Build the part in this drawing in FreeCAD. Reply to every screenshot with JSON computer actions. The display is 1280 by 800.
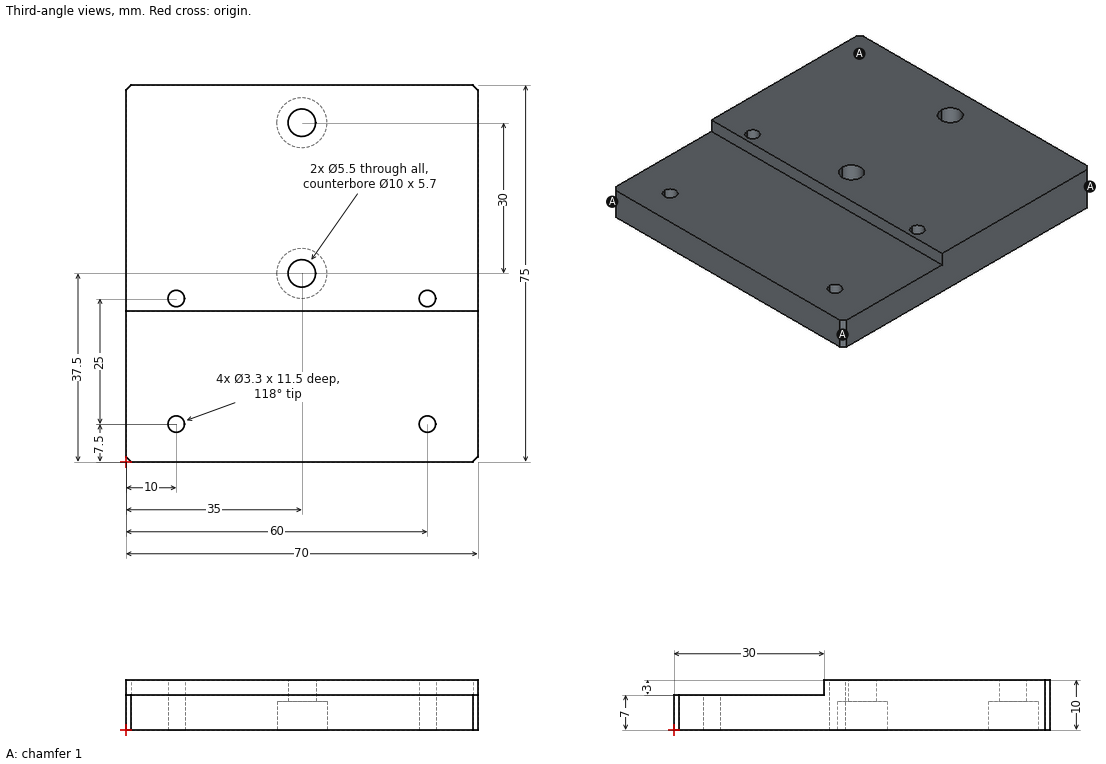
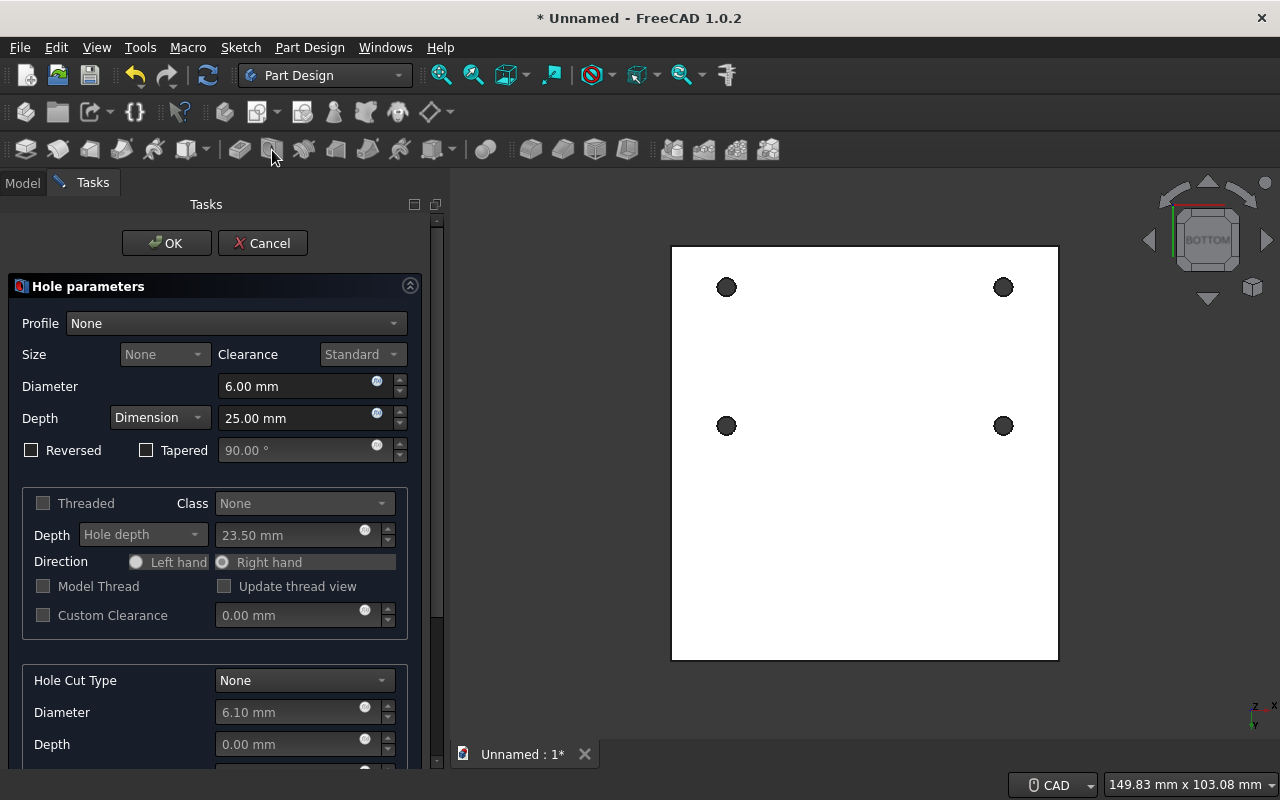
{"action": "triple_click", "coordinate": [305, 386]}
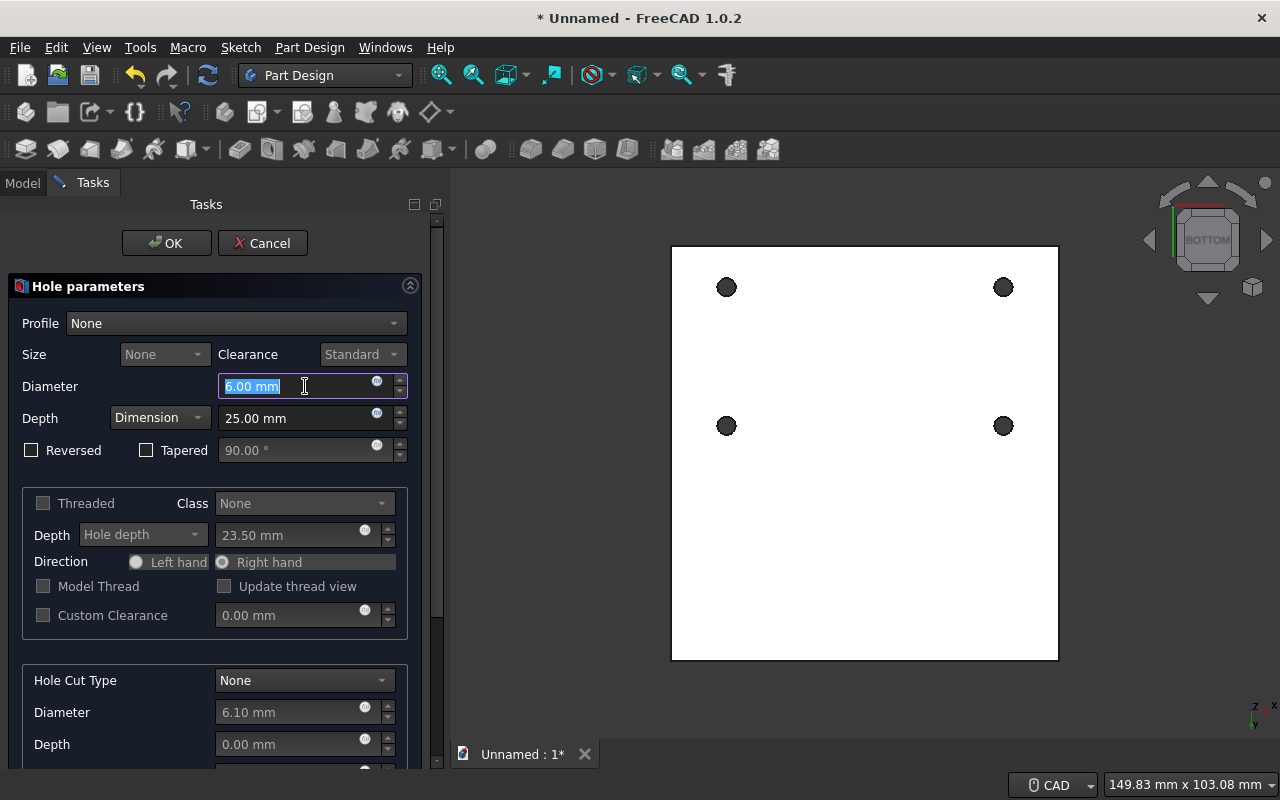
{"action": "type", "text": "5.5"}
{"action": "key", "text": "Tab"}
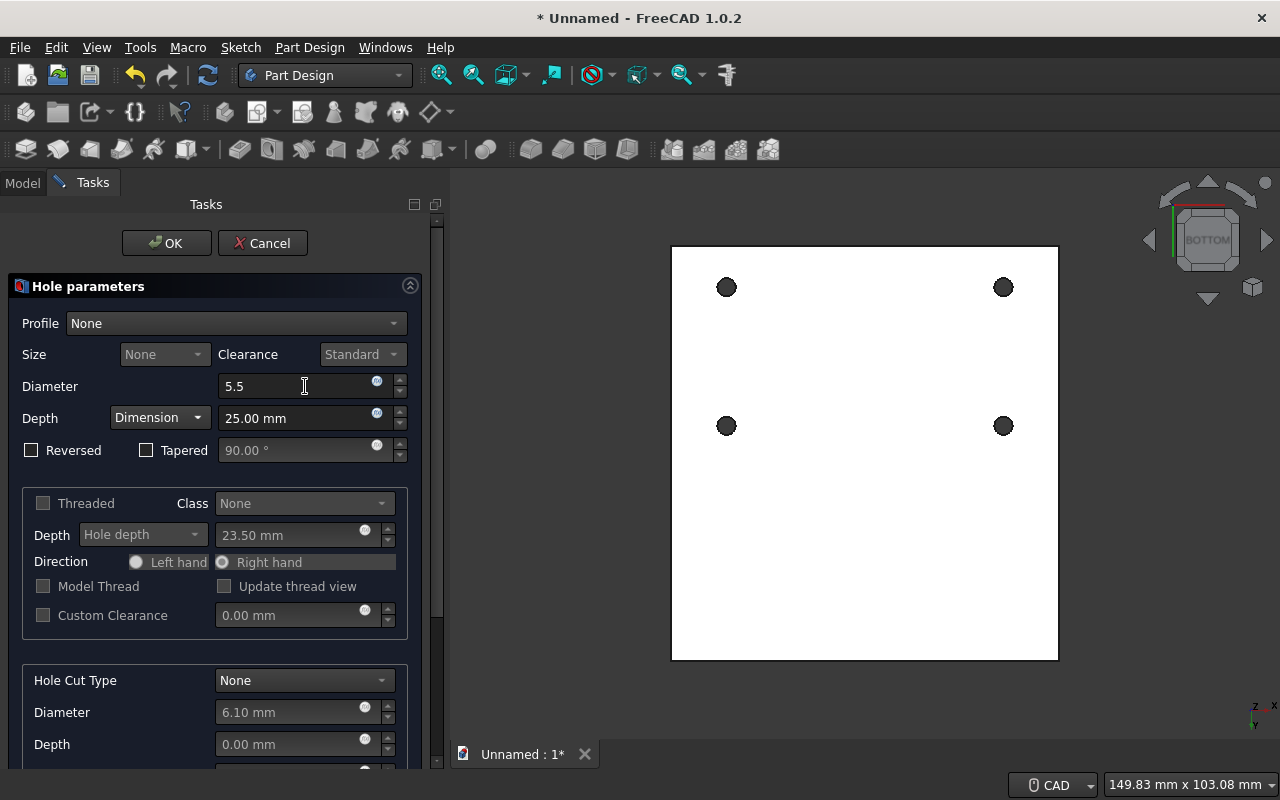
{"action": "left_click", "coordinate": [161, 418]}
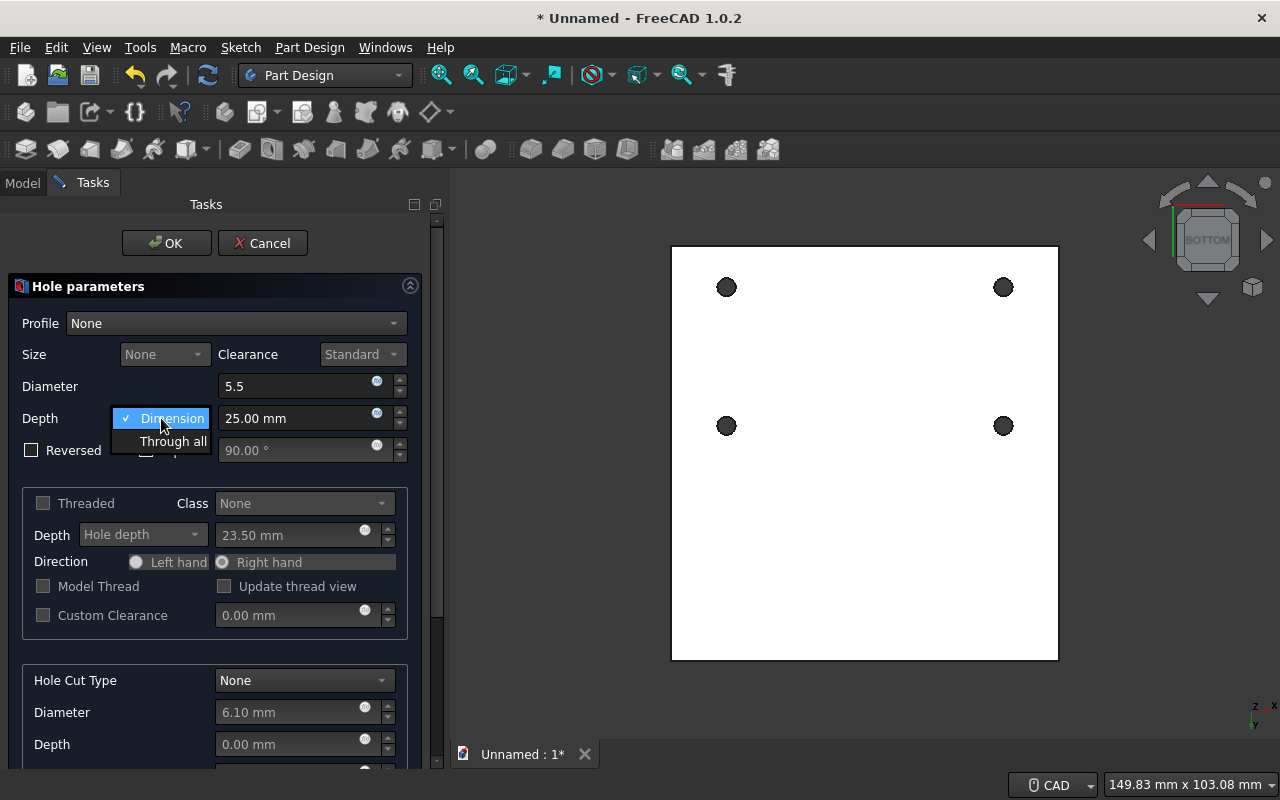
{"action": "left_click", "coordinate": [160, 442]}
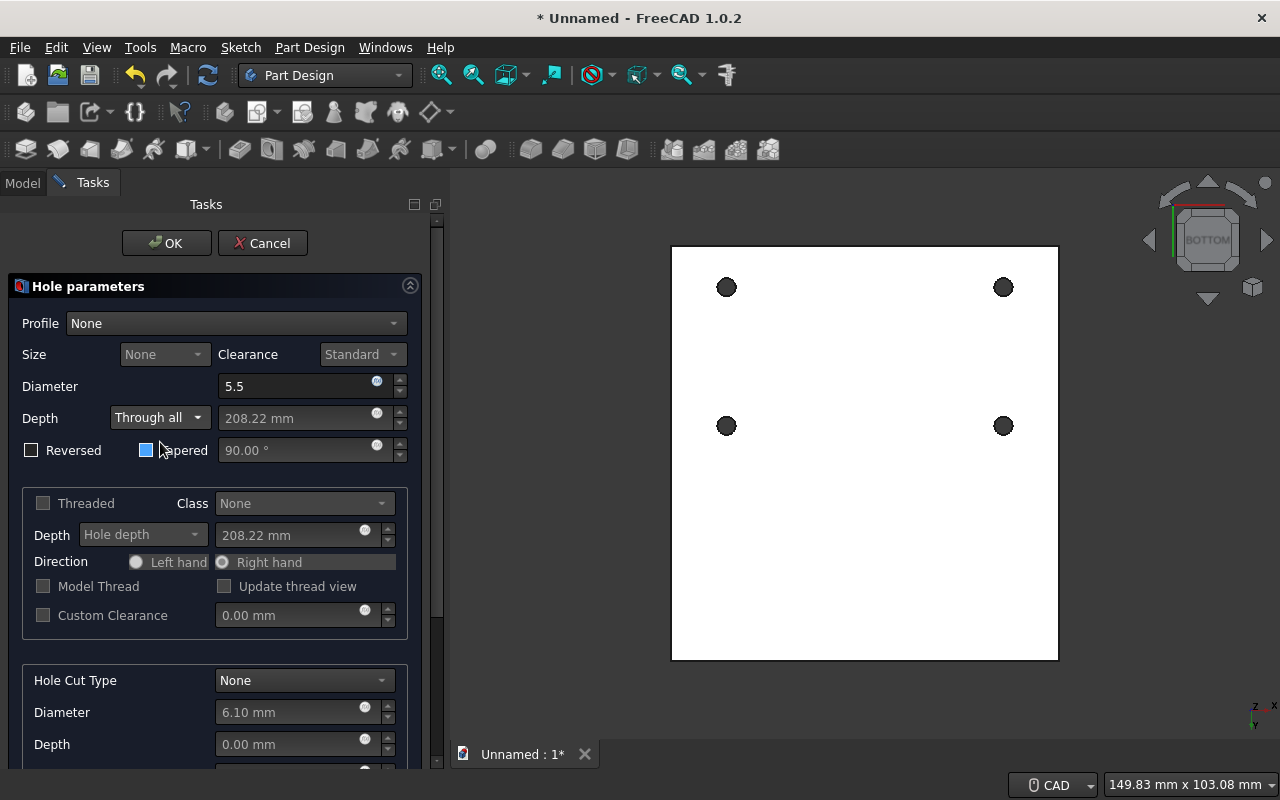
{"action": "left_click", "coordinate": [30, 450]}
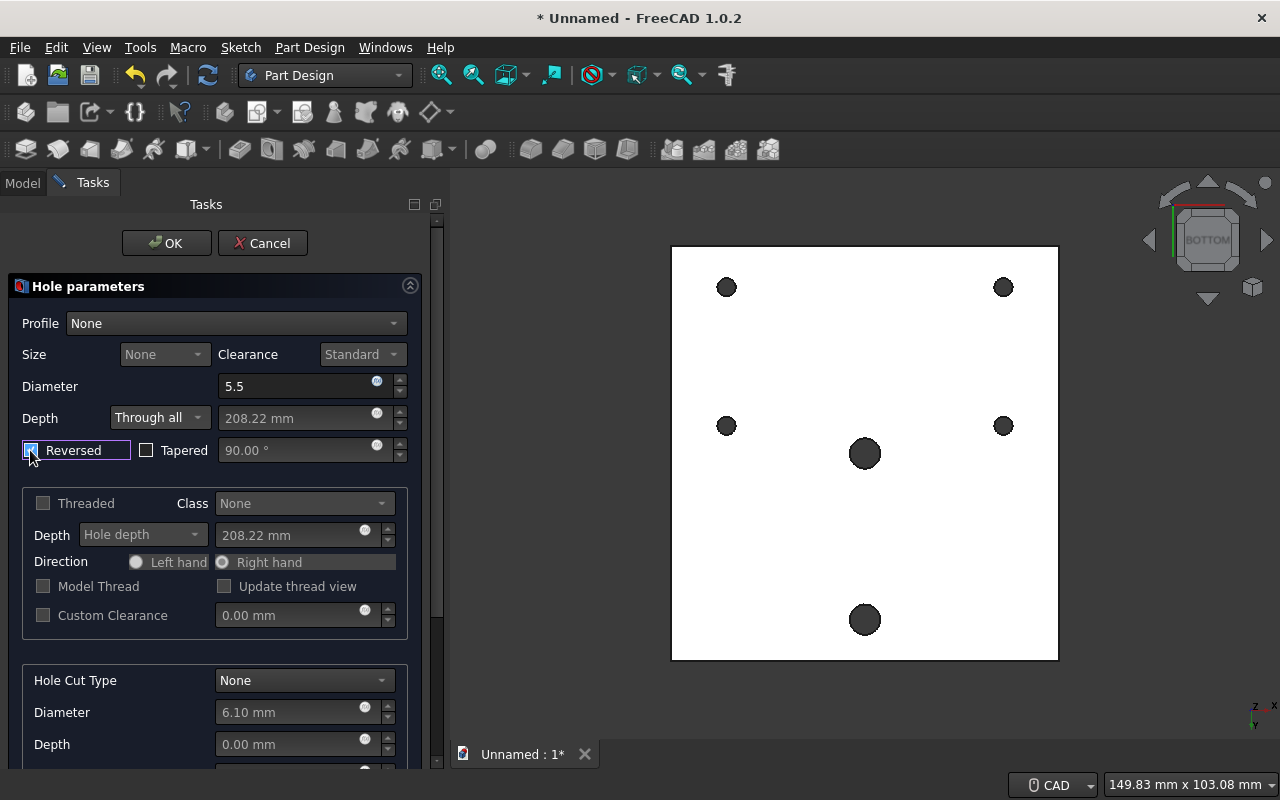
{"action": "left_click", "coordinate": [306, 680]}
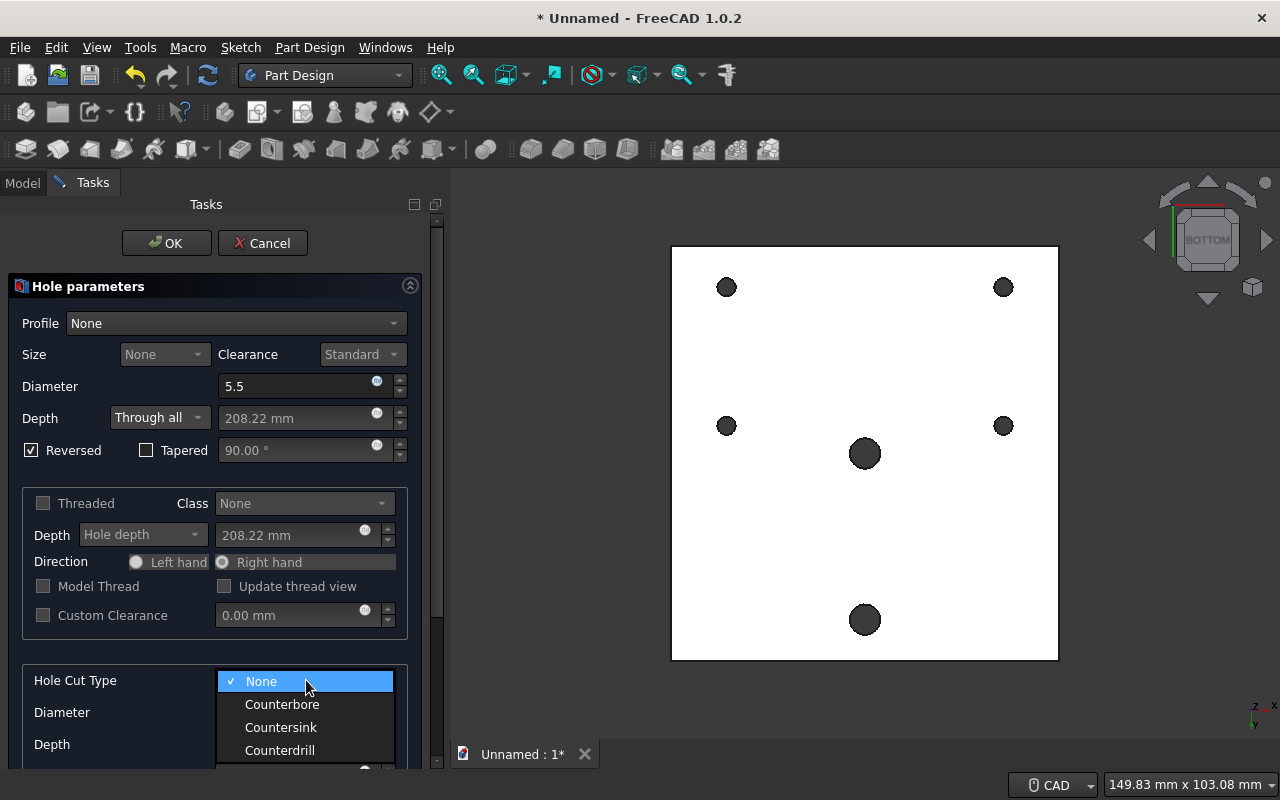
{"action": "left_click", "coordinate": [304, 704]}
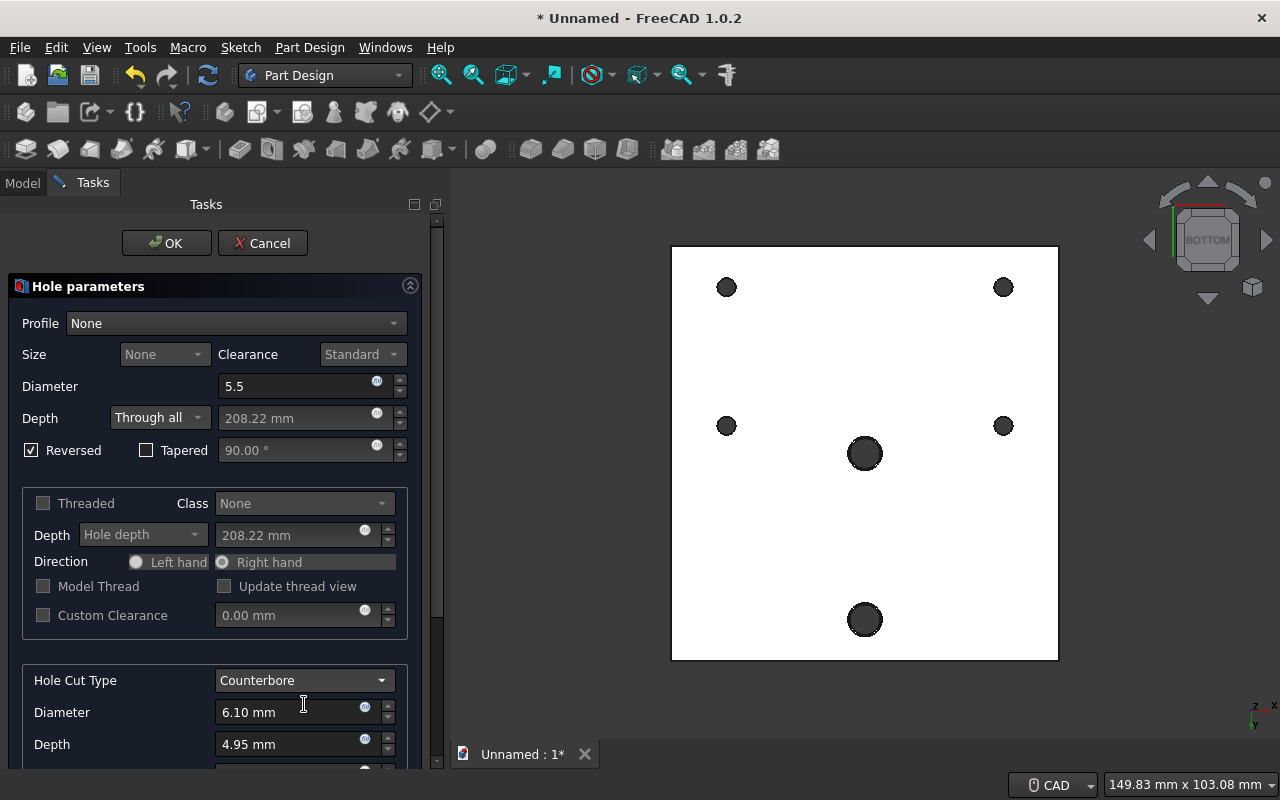
{"action": "triple_click", "coordinate": [298, 712]}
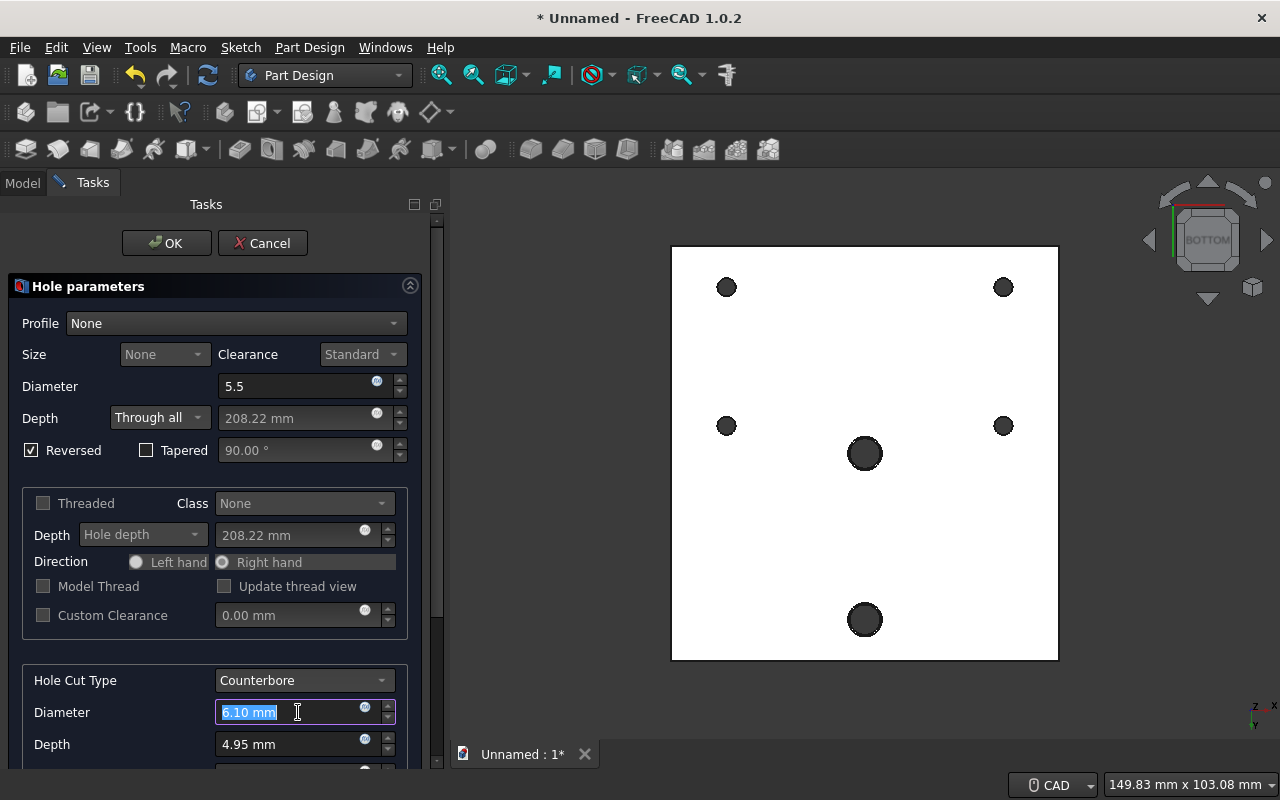
{"action": "type", "text": "10"}
{"action": "key", "text": "Tab"}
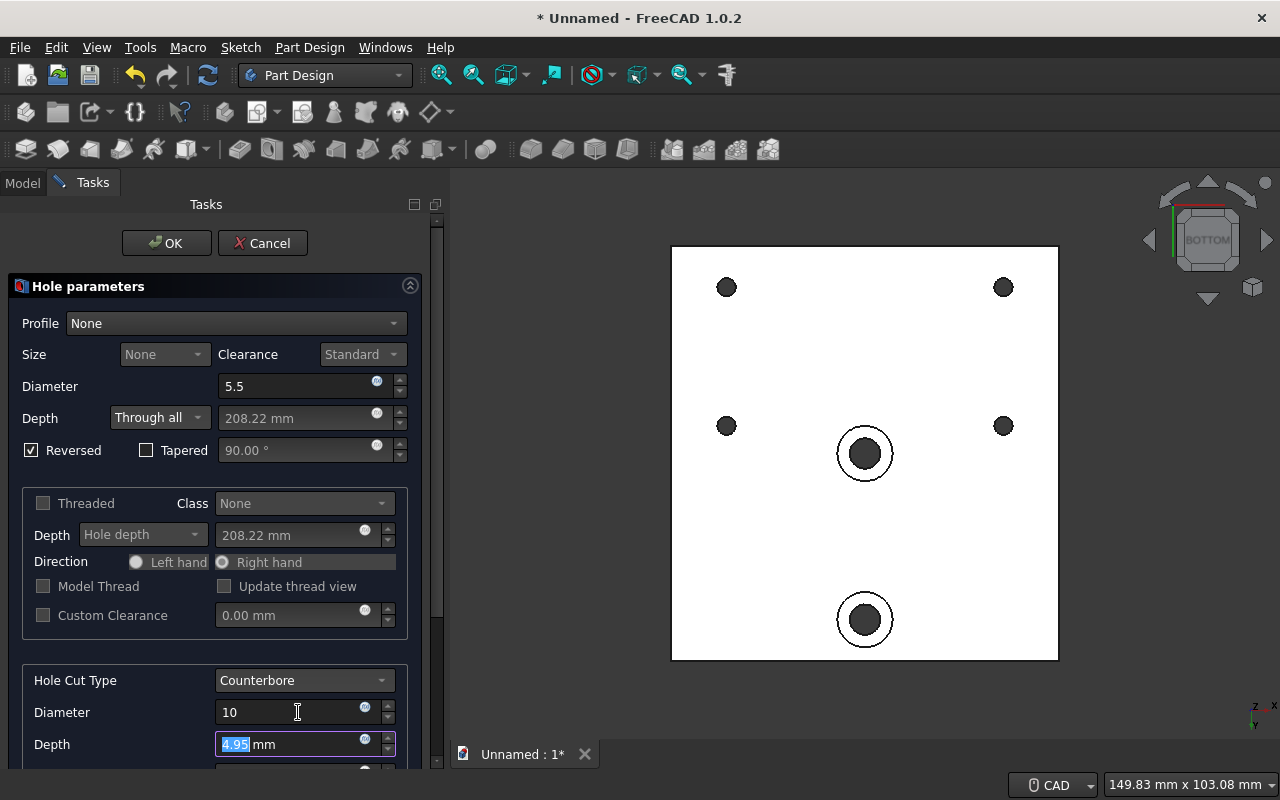
{"action": "type", "text": "5.7"}
{"action": "key", "text": "Tab"}